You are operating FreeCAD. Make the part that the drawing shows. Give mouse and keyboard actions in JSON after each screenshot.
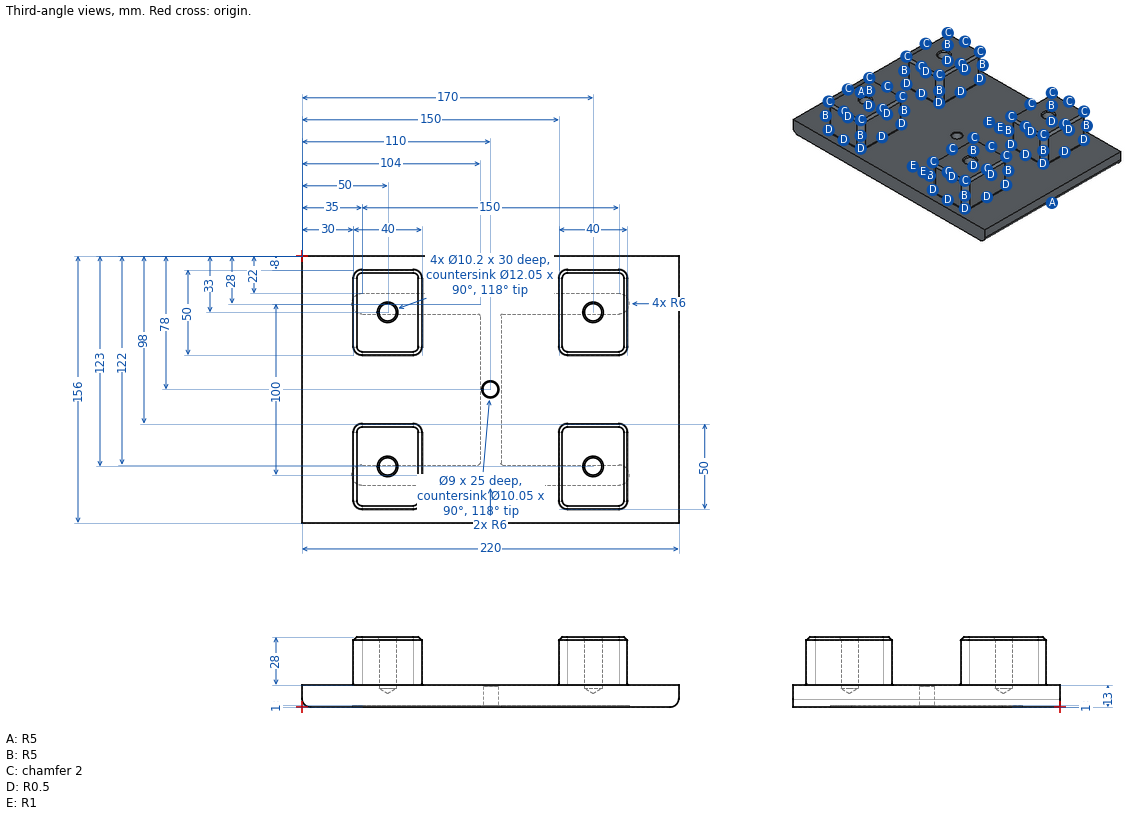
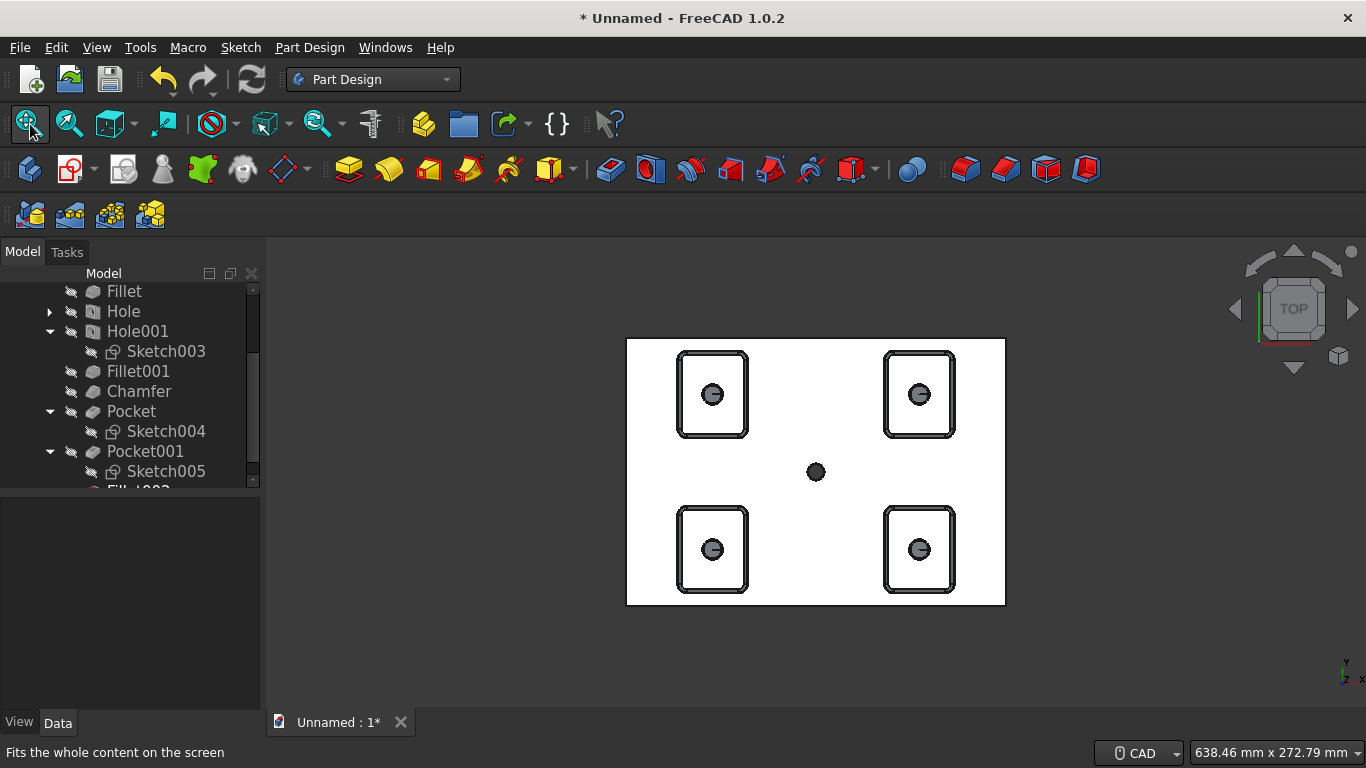
{"action": "scroll", "coordinate": [806, 547], "scroll_direction": "up", "scroll_amount": 15}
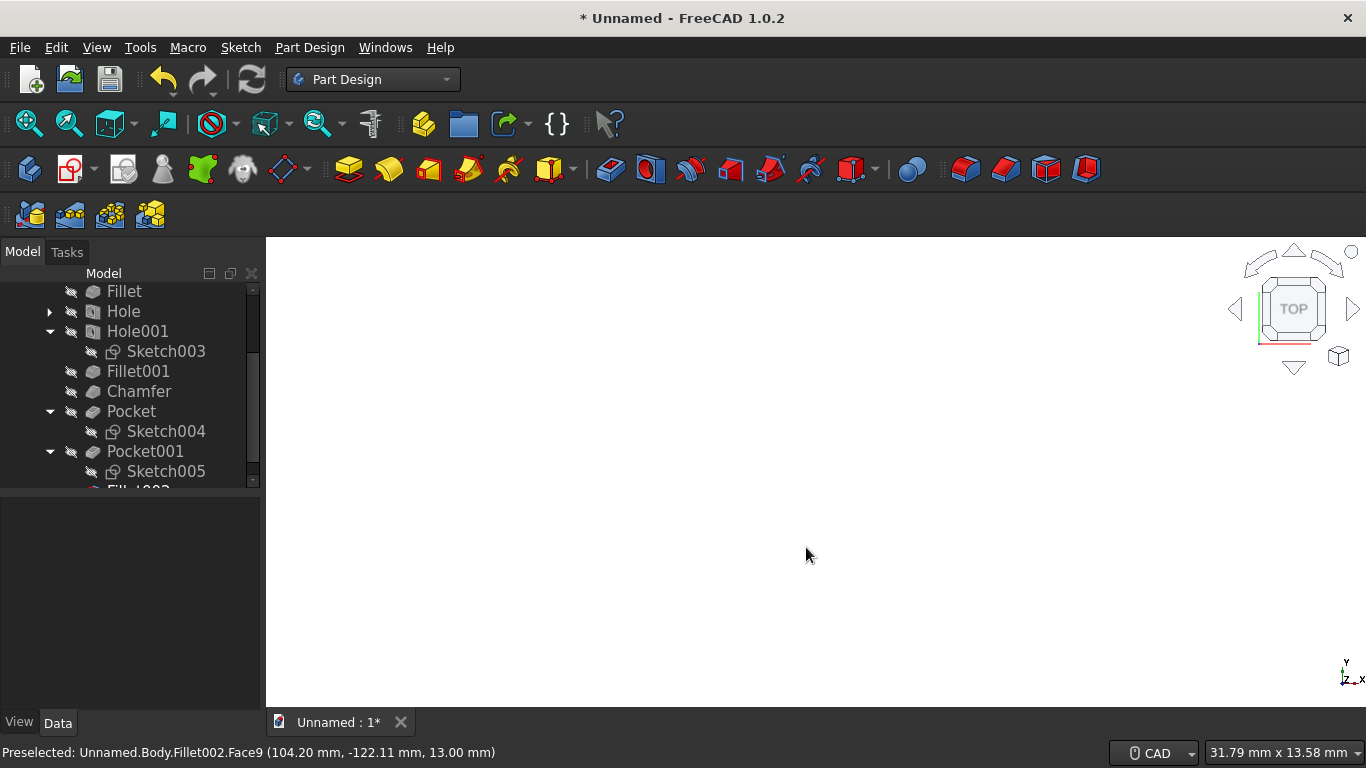
{"action": "key", "text": "v f"}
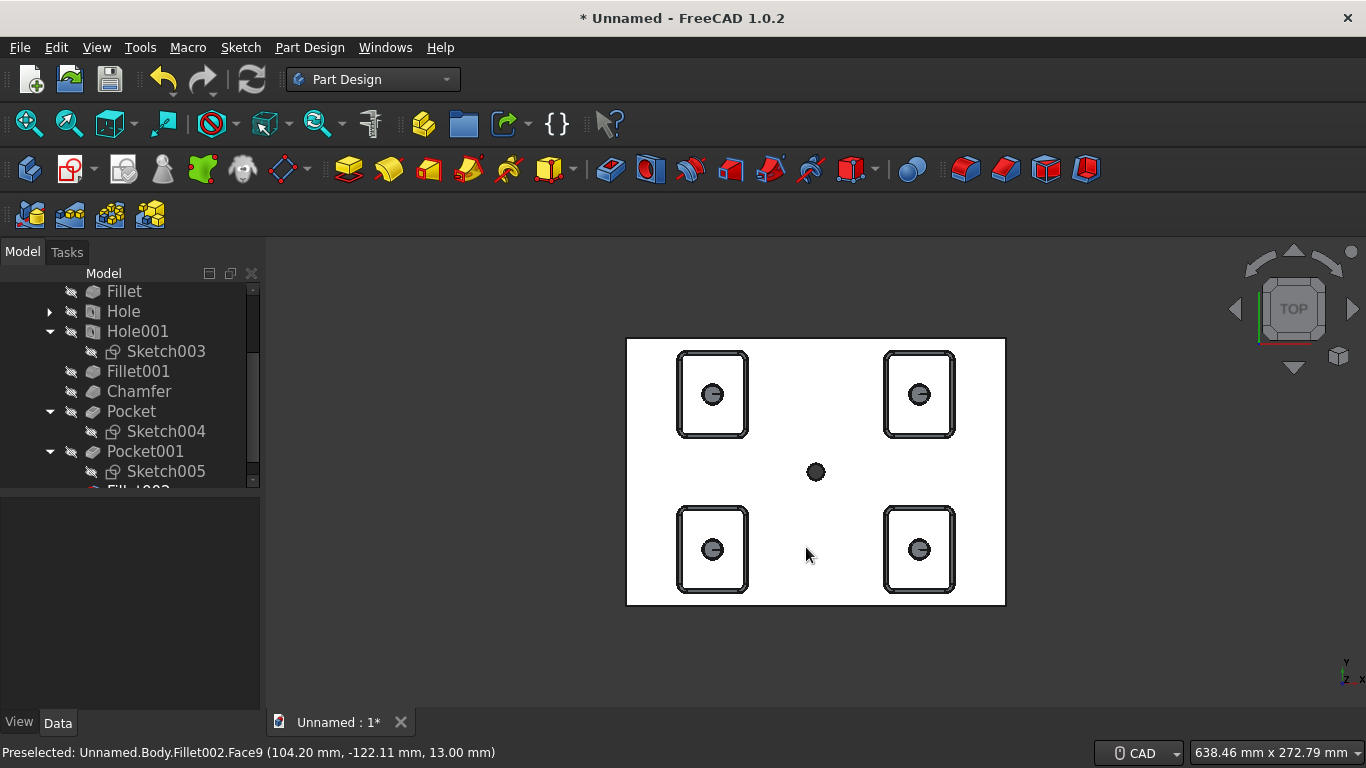
{"action": "key", "text": "1"}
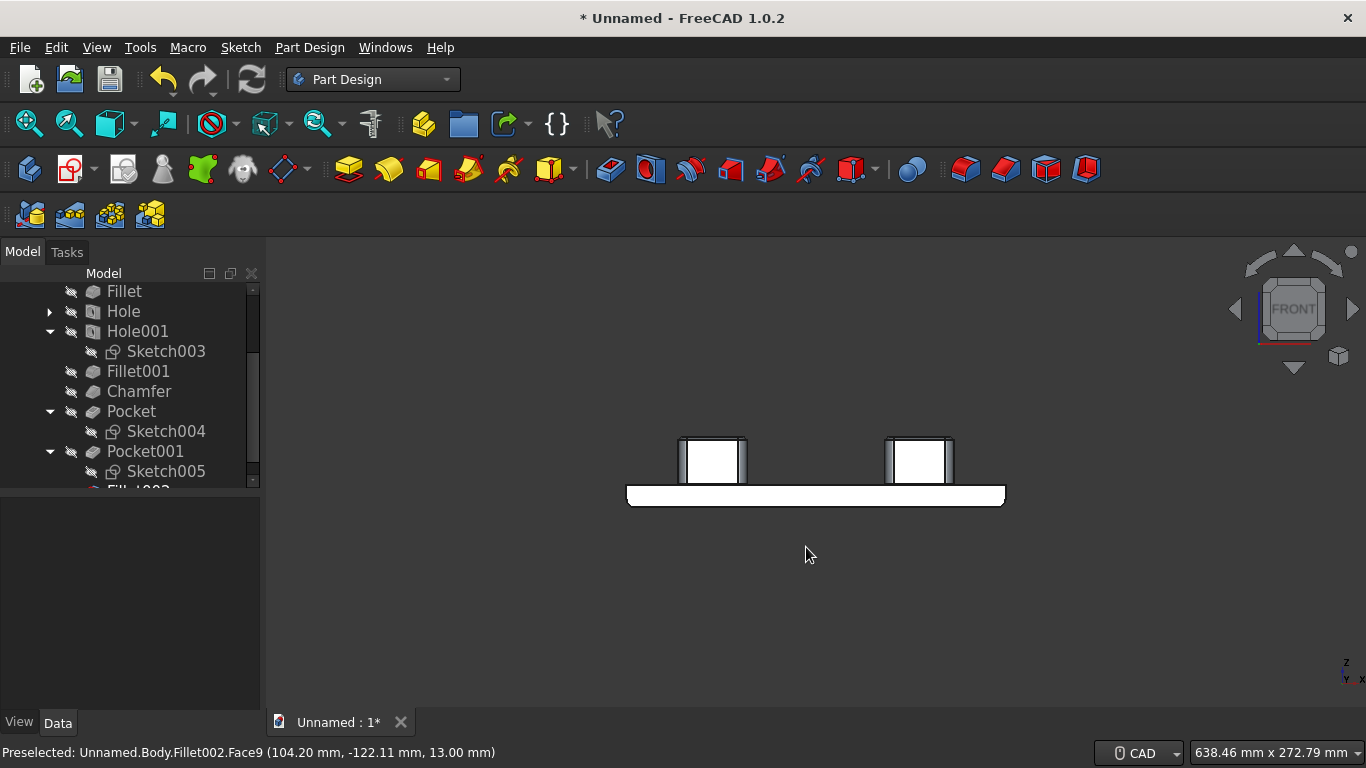
{"action": "key", "text": "v f"}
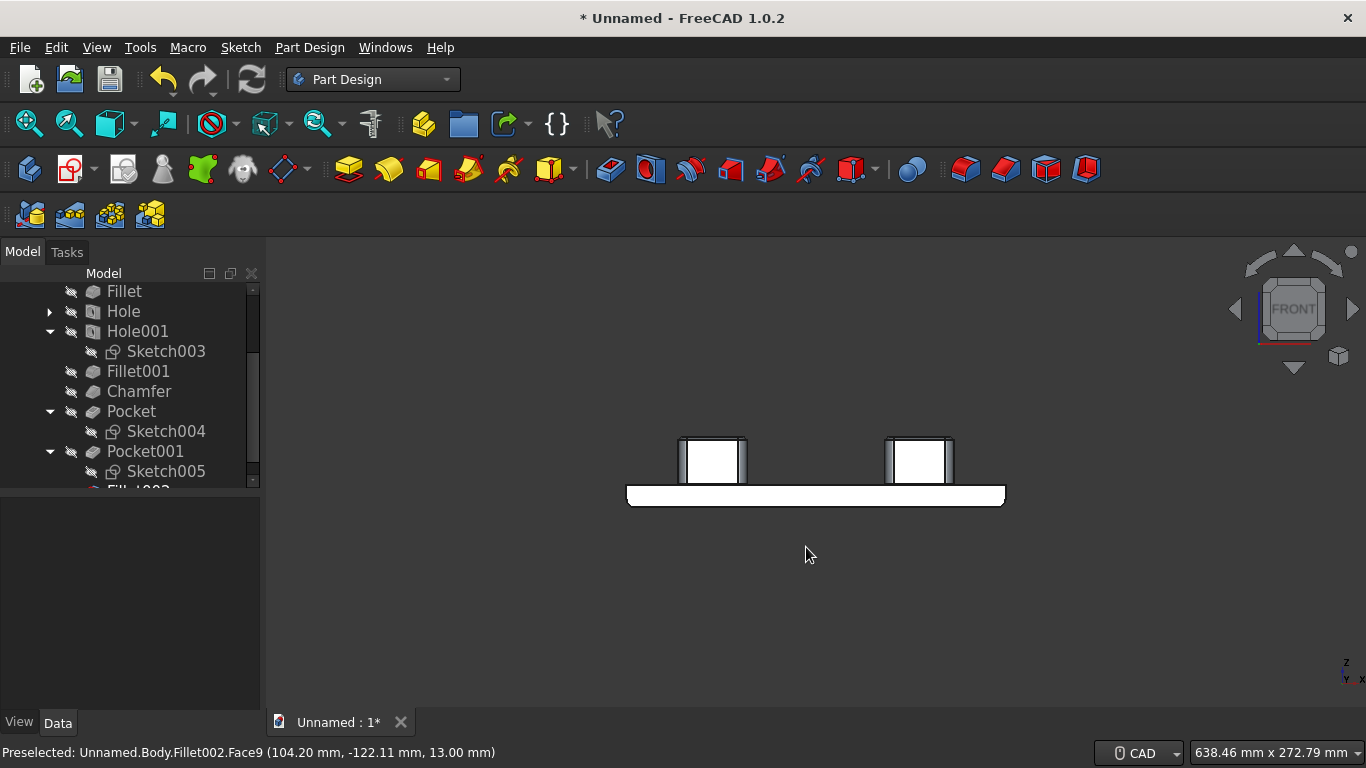
{"action": "scroll", "coordinate": [806, 505], "scroll_direction": "up", "scroll_amount": 15}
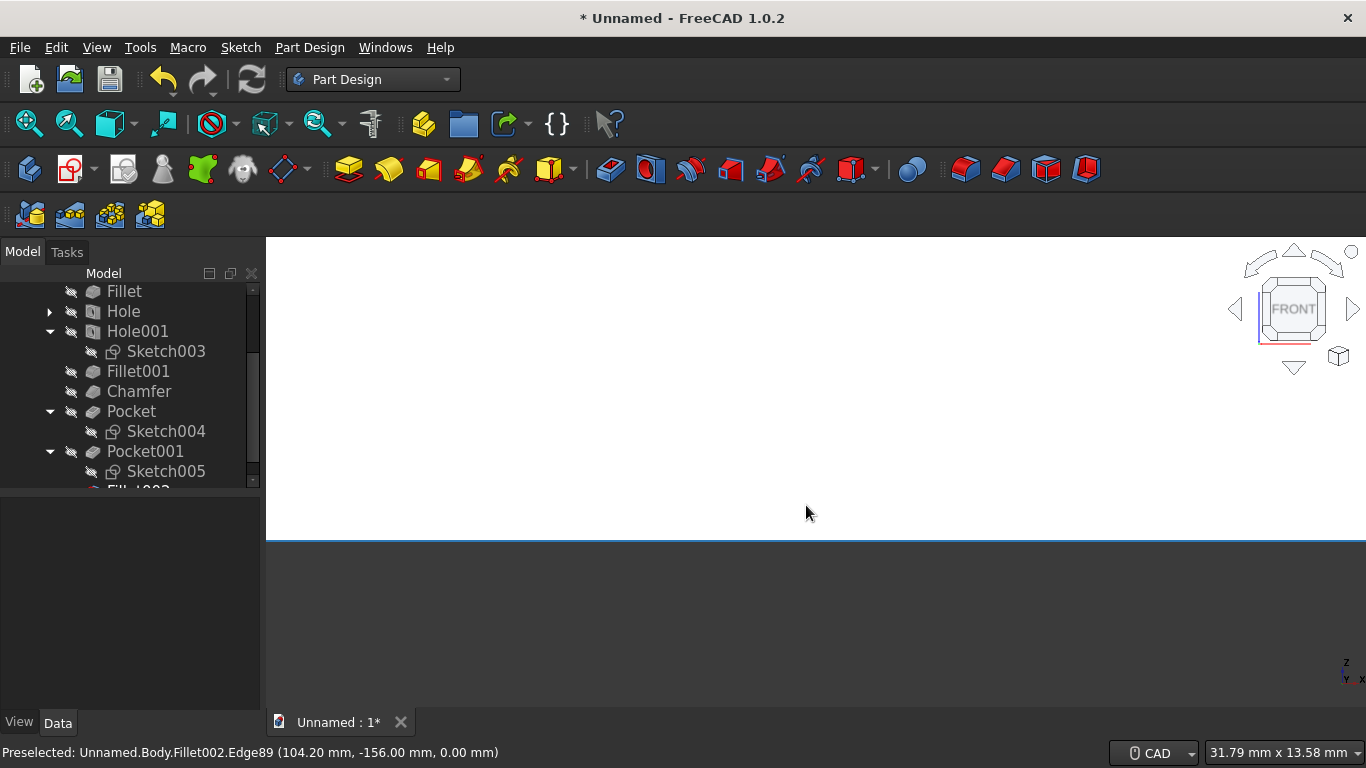
{"action": "key", "text": "v f"}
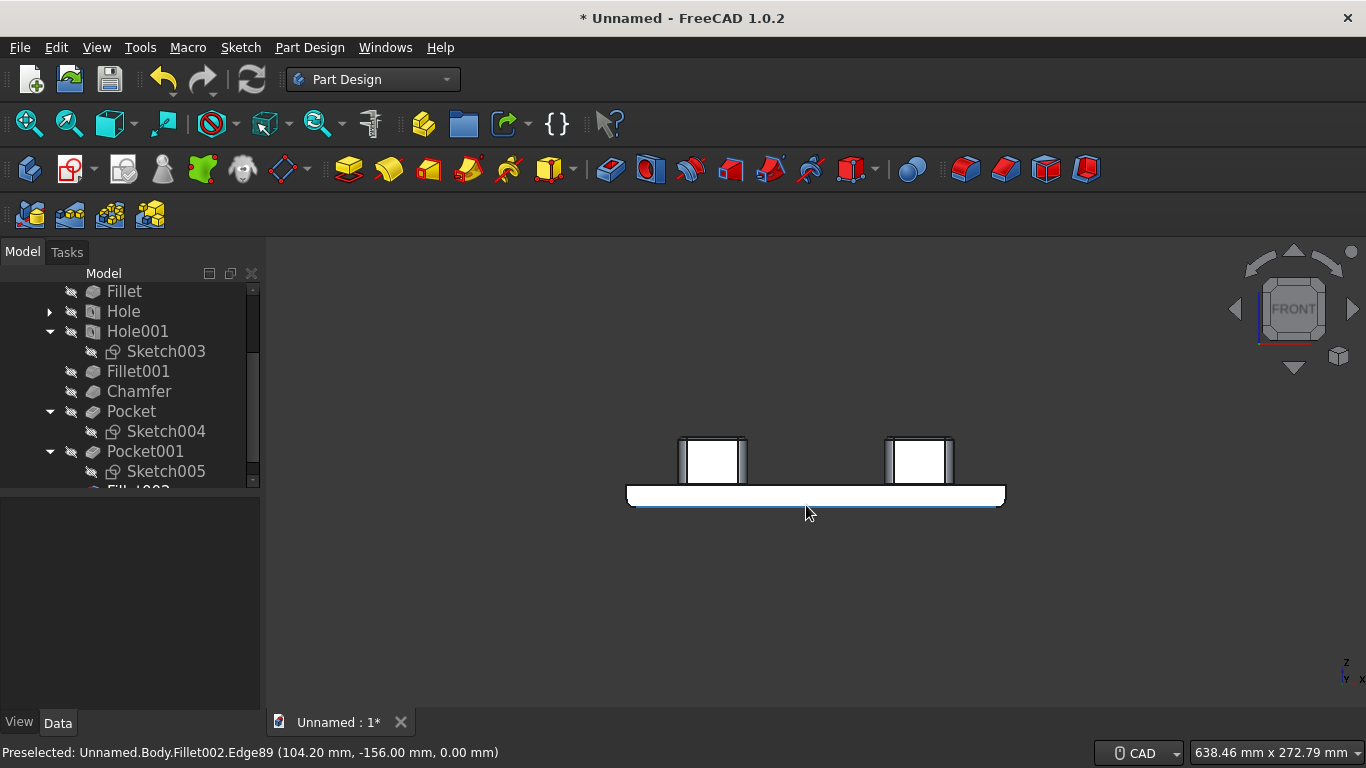
{"action": "key", "text": "3"}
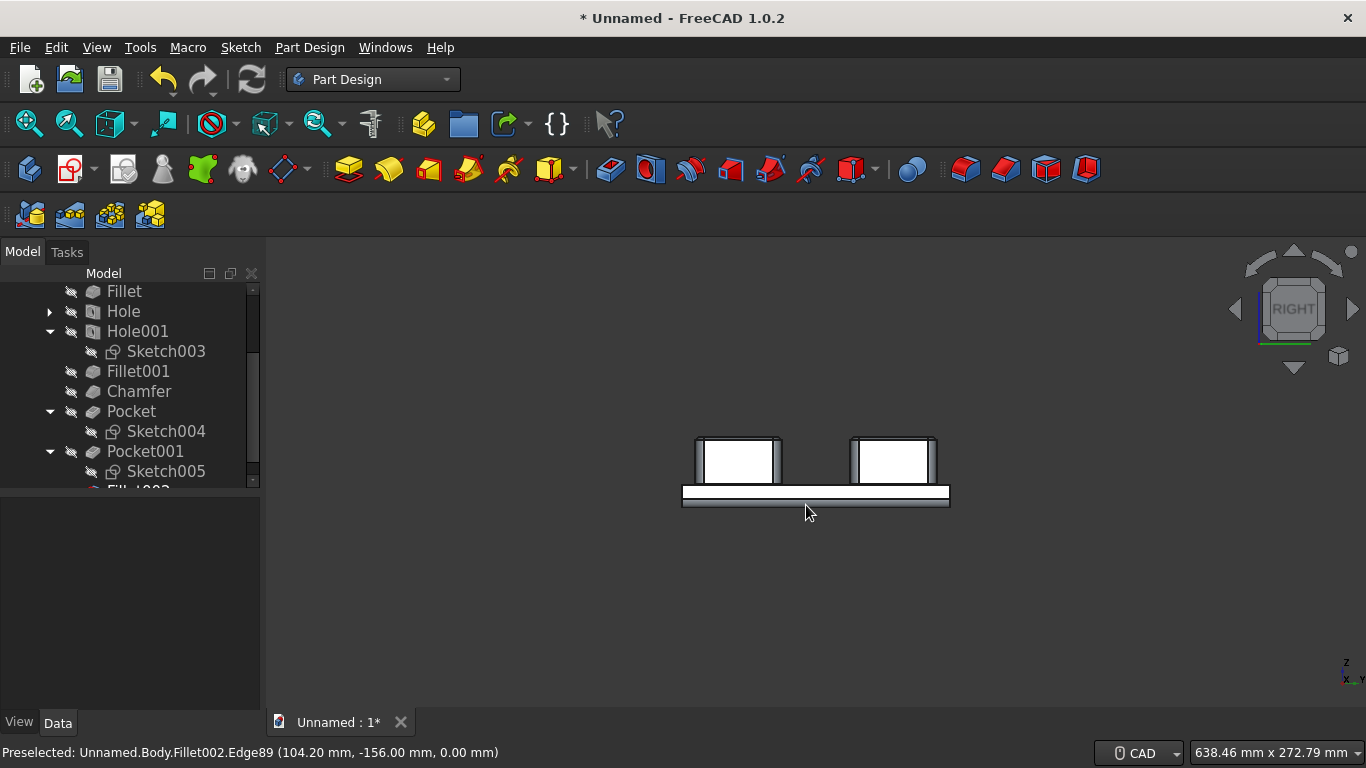
{"action": "key", "text": "v f"}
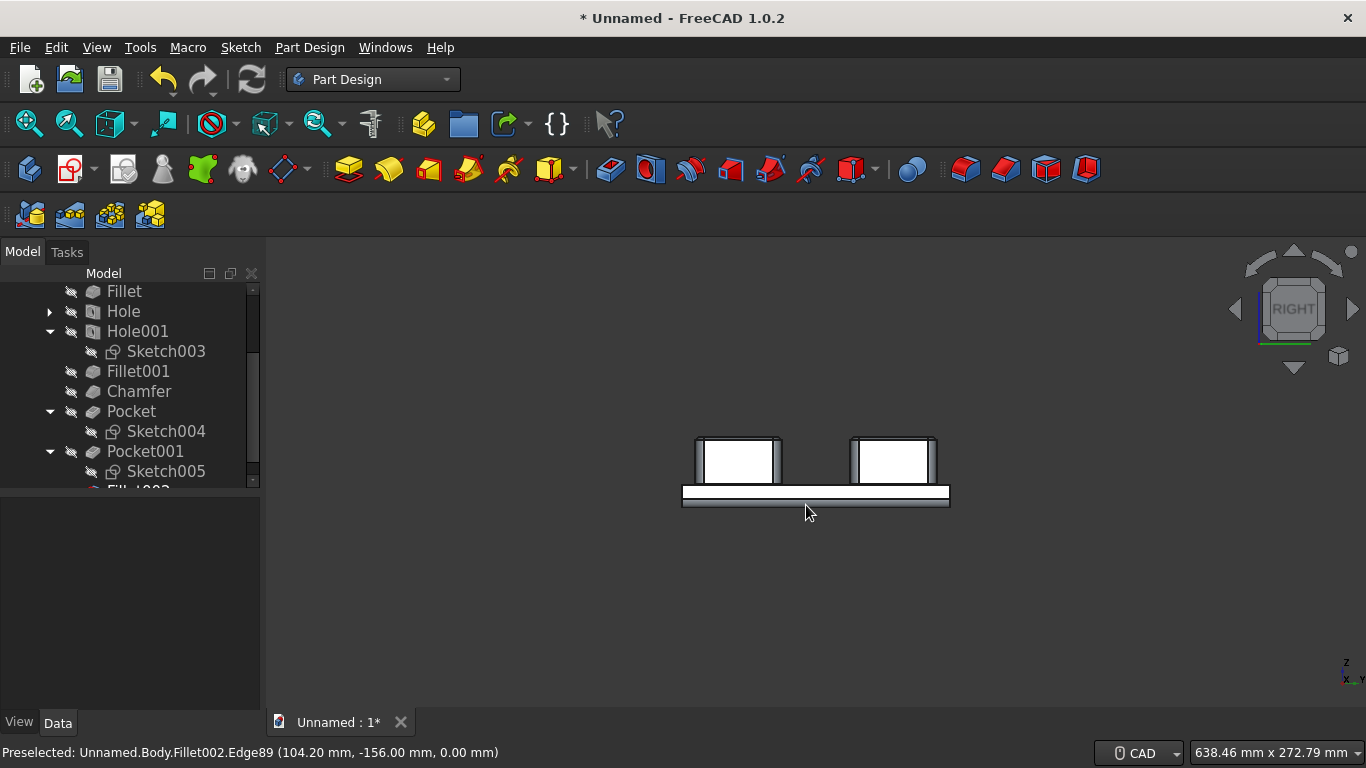
{"action": "scroll", "coordinate": [740, 505], "scroll_direction": "up", "scroll_amount": 15}